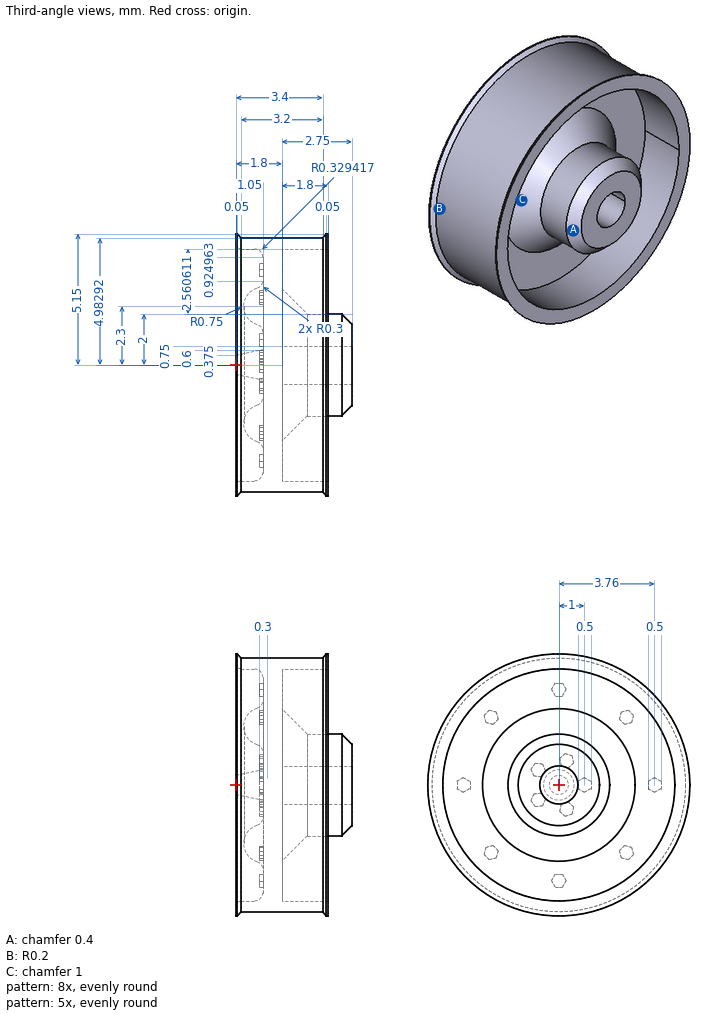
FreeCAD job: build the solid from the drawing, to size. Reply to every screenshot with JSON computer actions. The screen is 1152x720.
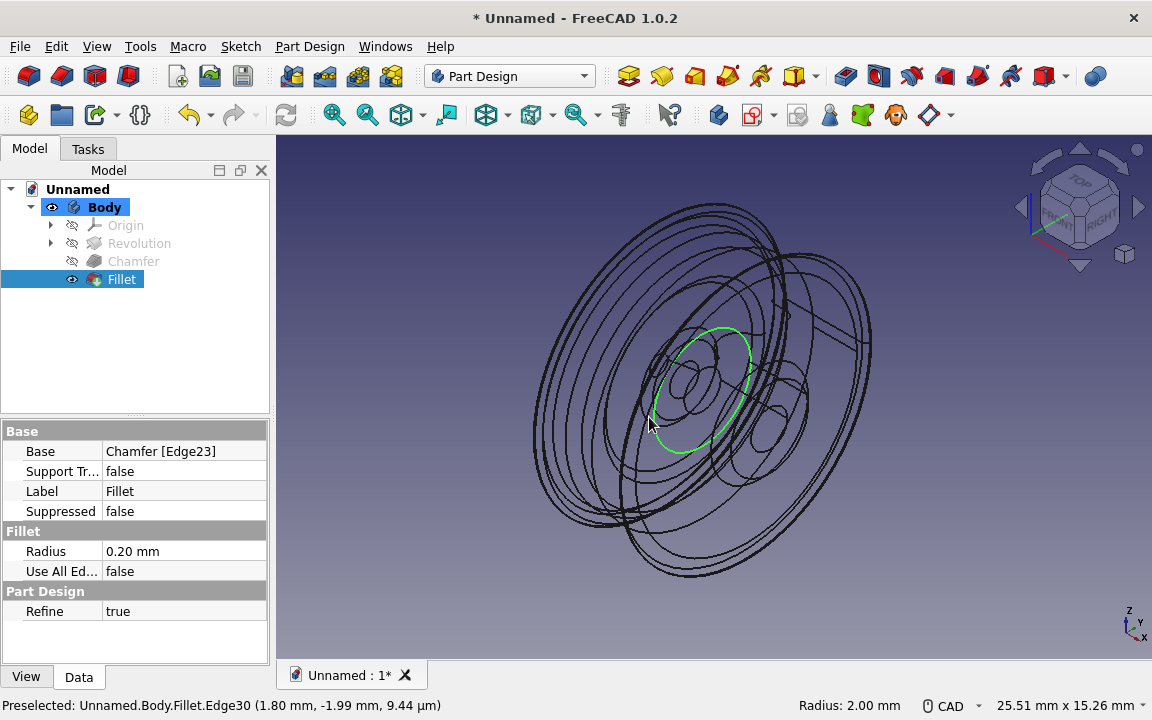
{"action": "key", "text": "v 1"}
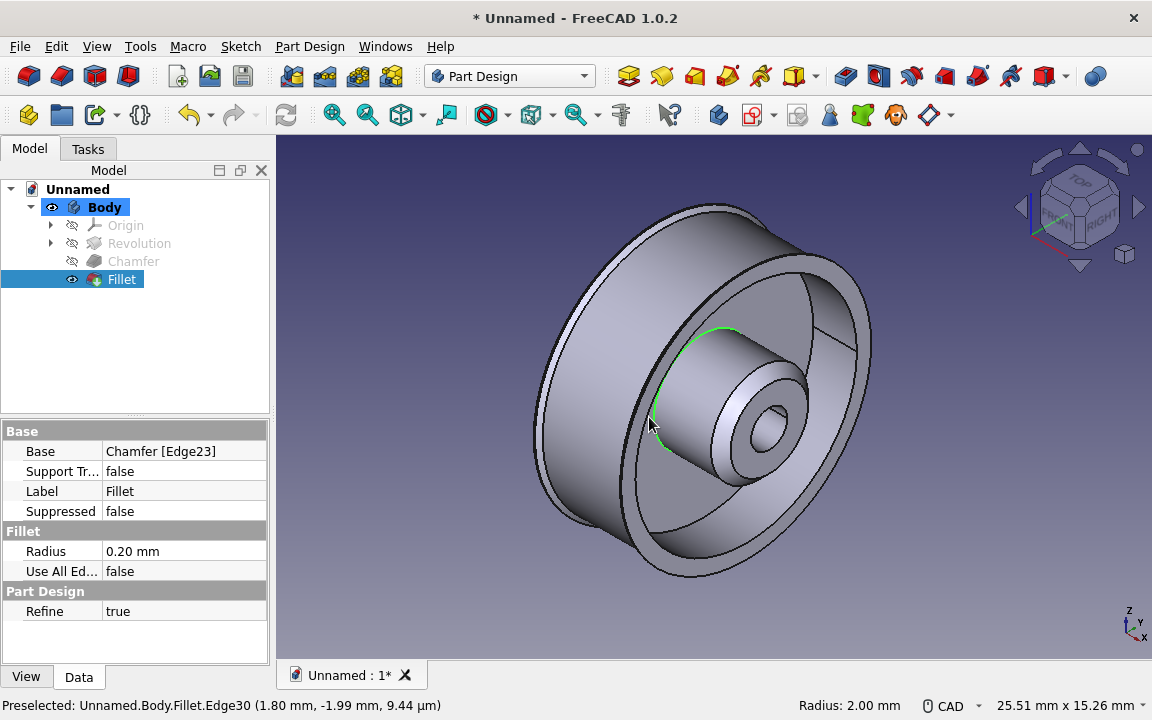
{"action": "left_click", "coordinate": [62, 76]}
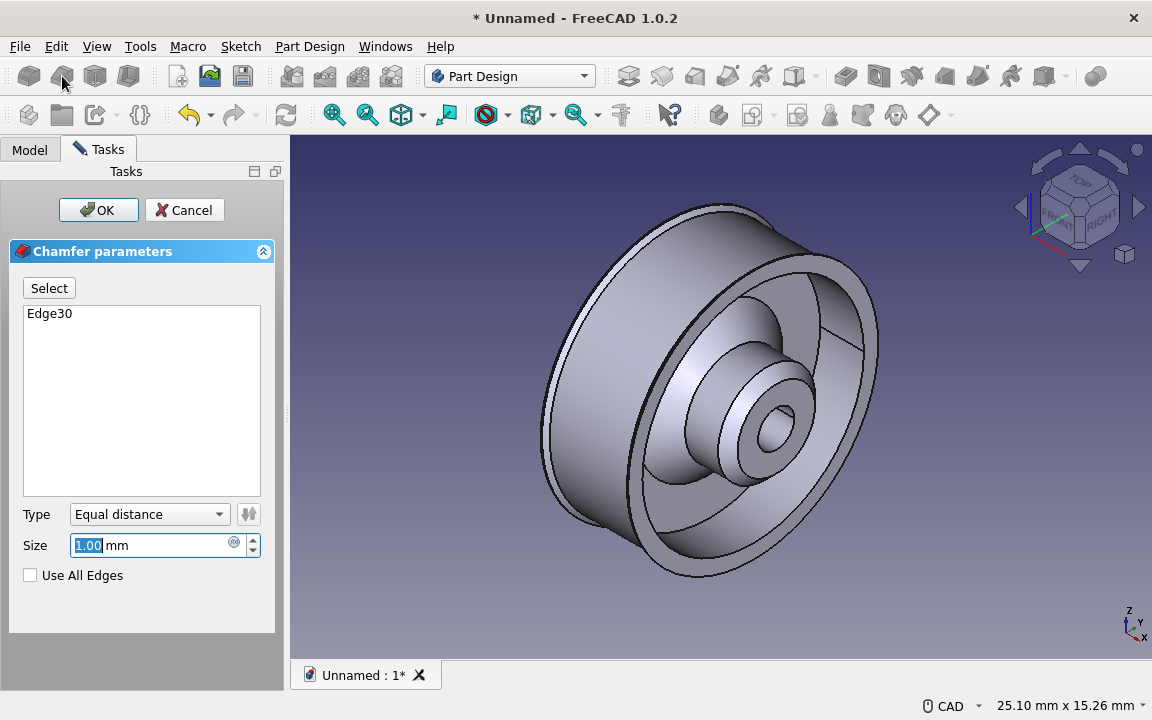
{"action": "type", "text": "1"}
{"action": "key", "text": "Tab"}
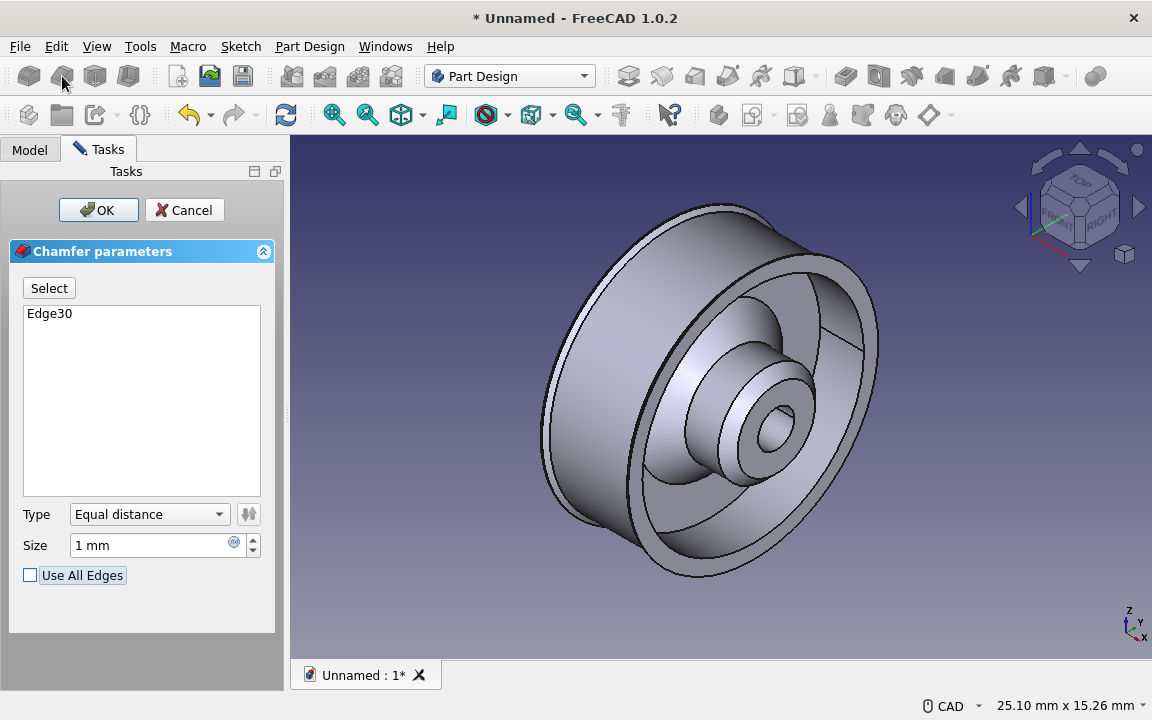
{"action": "left_click", "coordinate": [99, 210]}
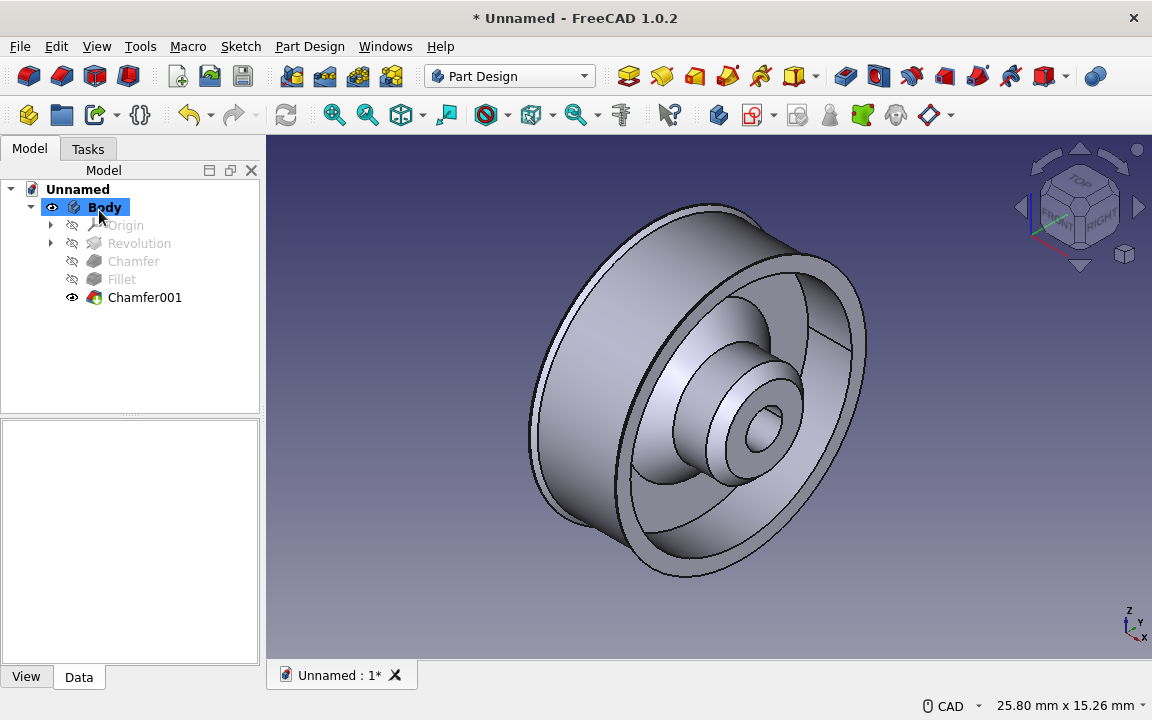
{"action": "key", "text": "6"}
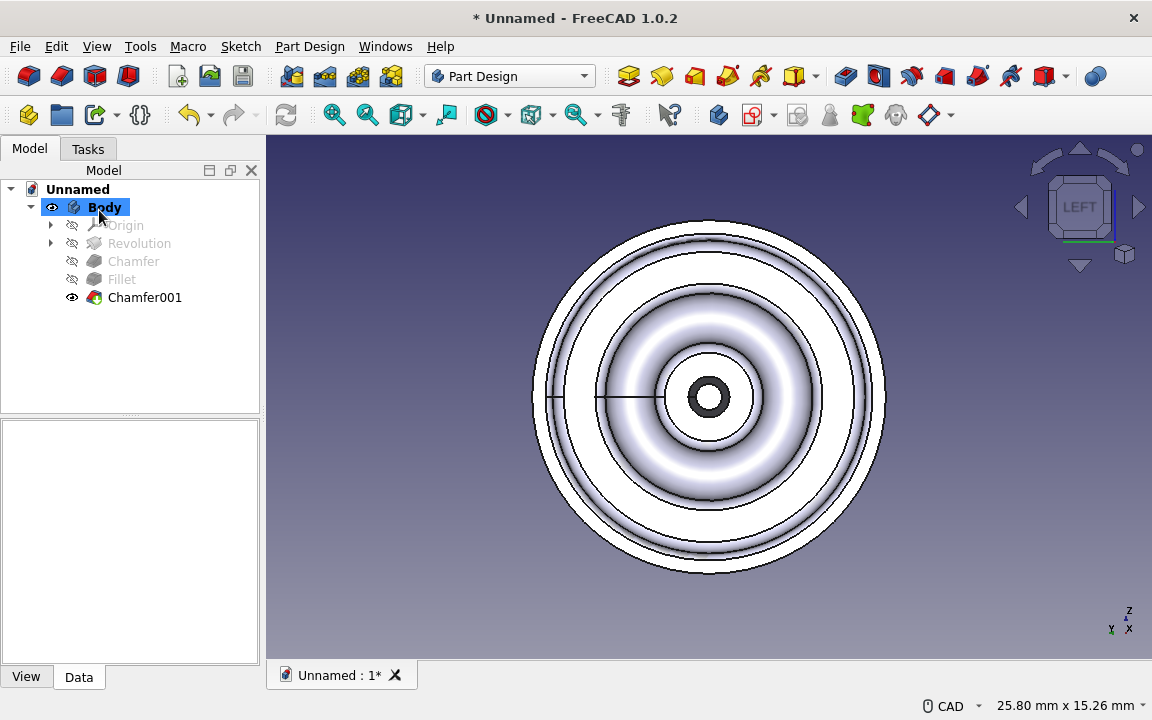
{"action": "left_click", "coordinate": [751, 271]}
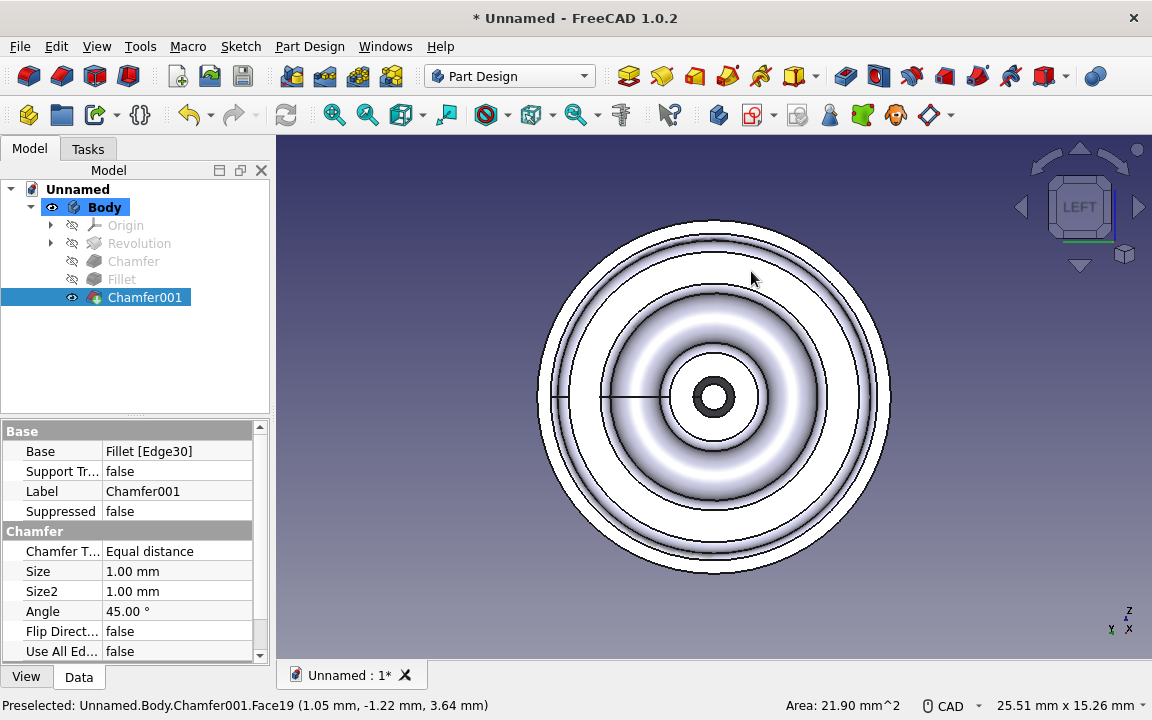
{"action": "left_click", "coordinate": [752, 116]}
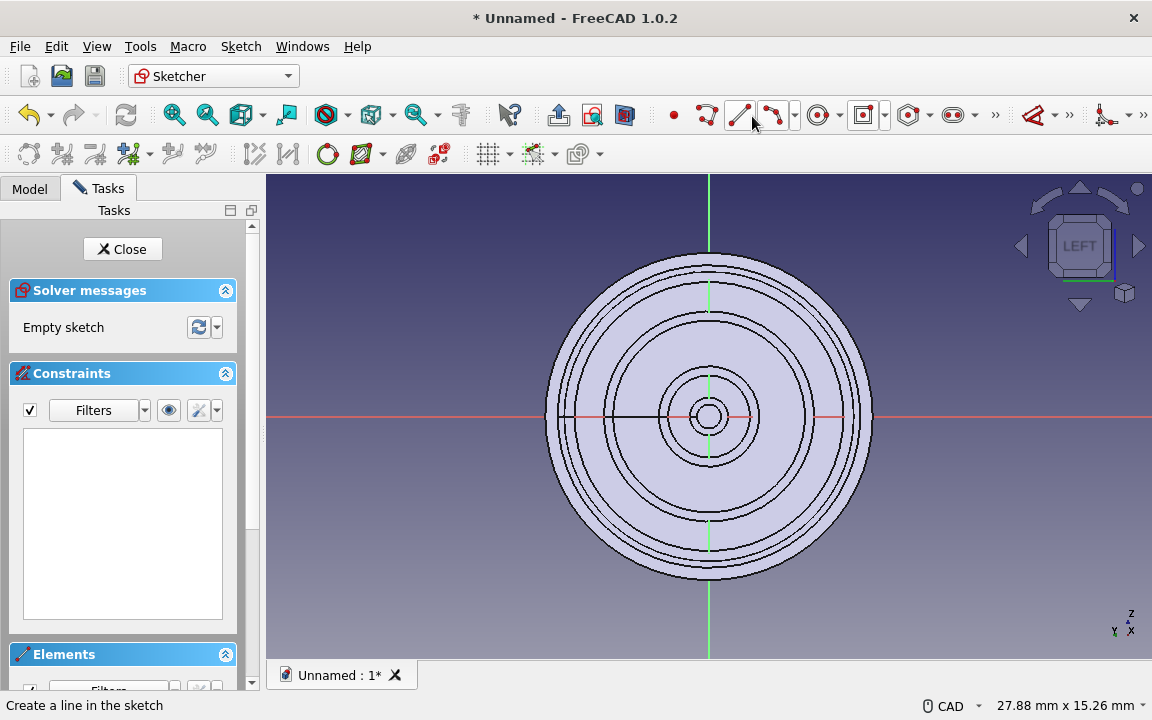
{"action": "left_click", "coordinate": [625, 116]}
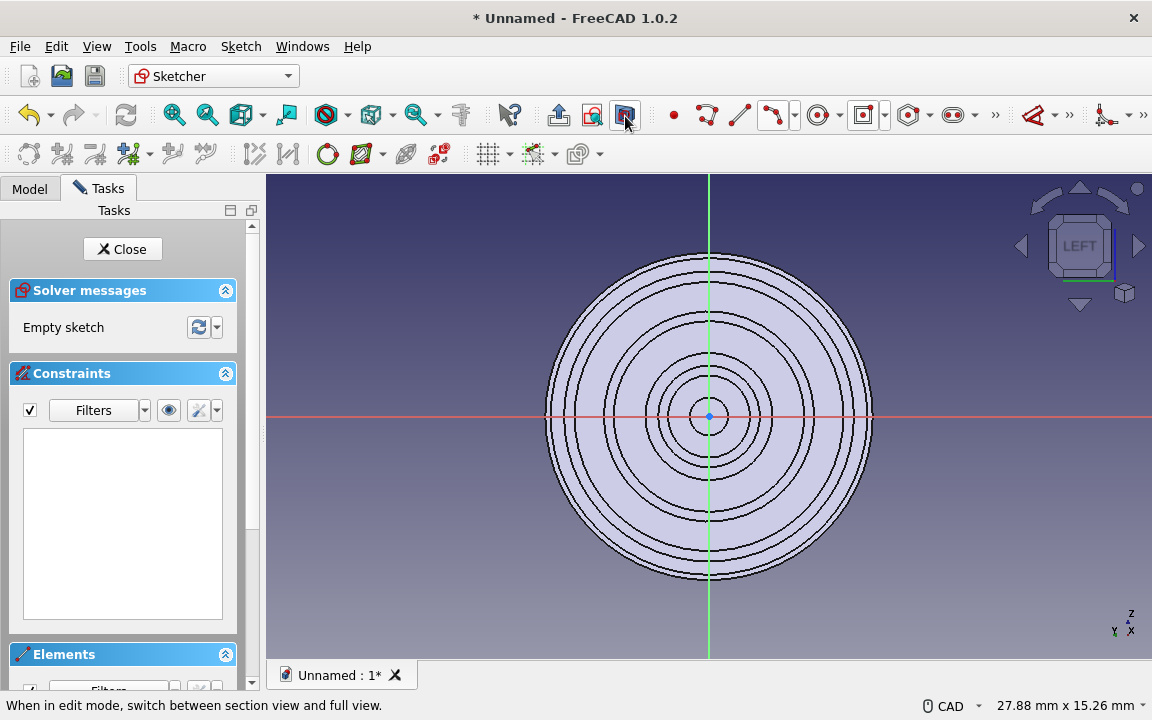
{"action": "scroll", "coordinate": [586, 416], "scroll_direction": "up", "scroll_amount": 14}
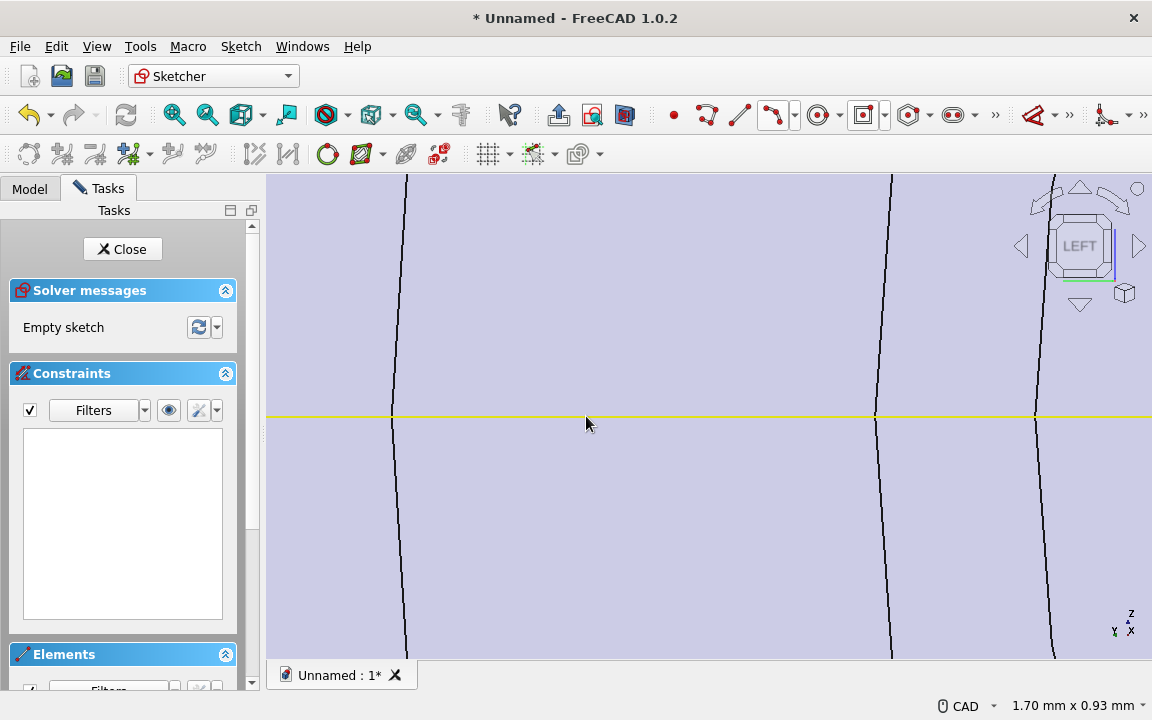
{"action": "left_click", "coordinate": [908, 116]}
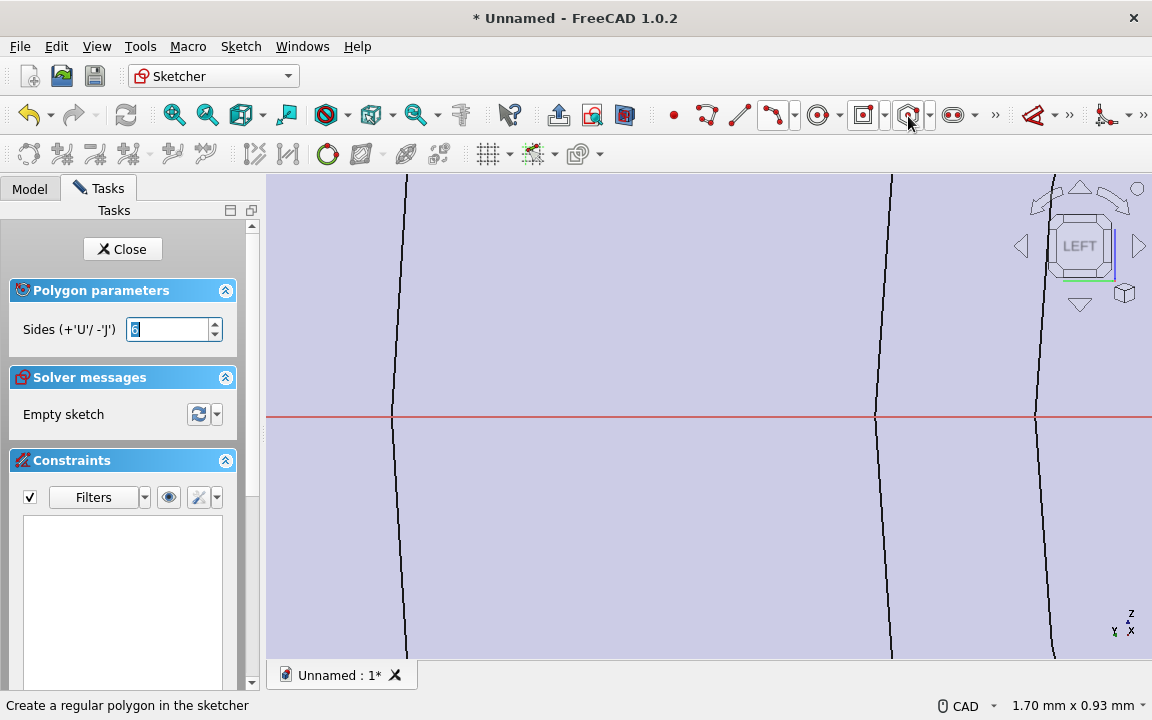
{"action": "left_click", "coordinate": [638, 416]}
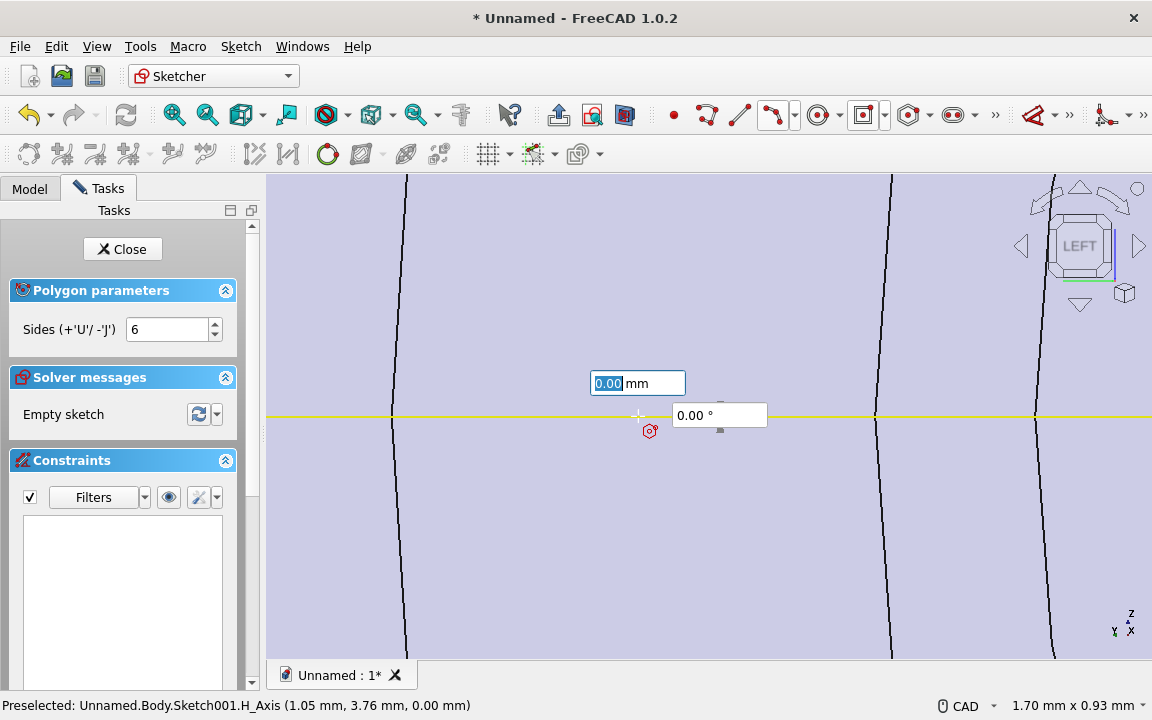
{"action": "left_click", "coordinate": [638, 266]}
{"action": "key", "text": "Escape"}